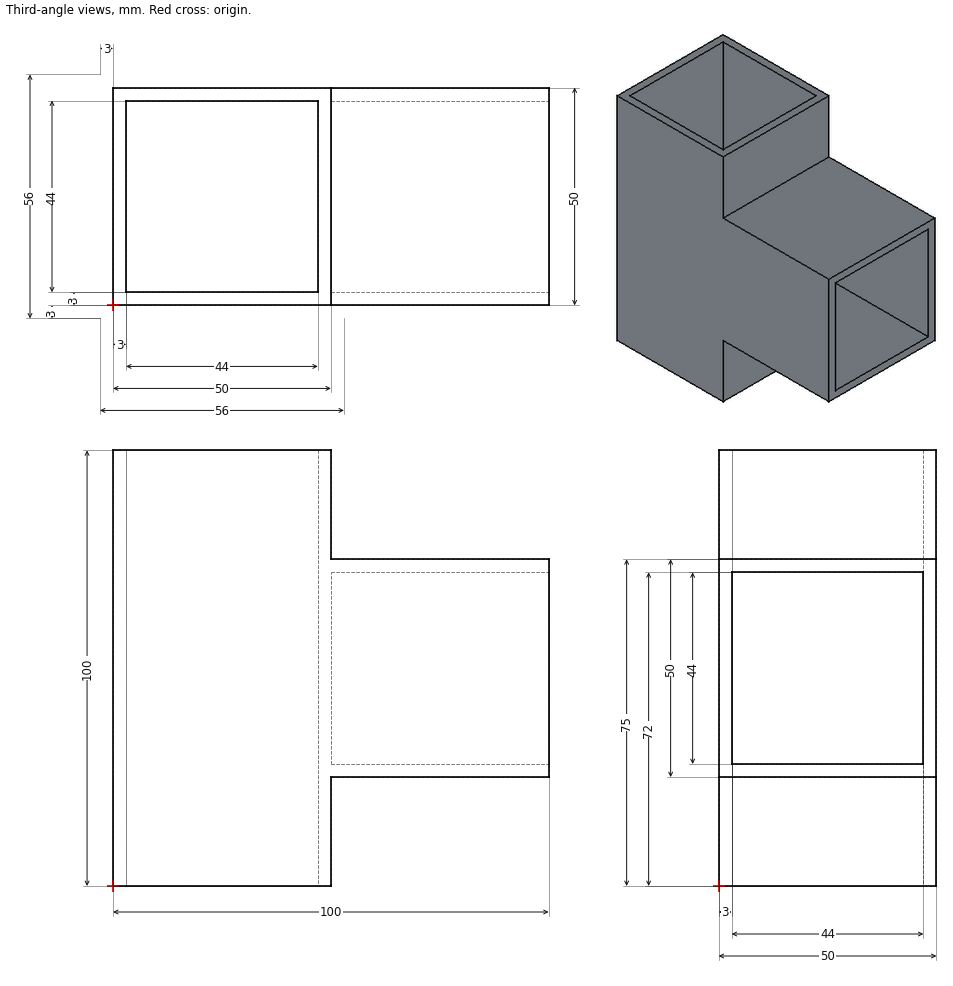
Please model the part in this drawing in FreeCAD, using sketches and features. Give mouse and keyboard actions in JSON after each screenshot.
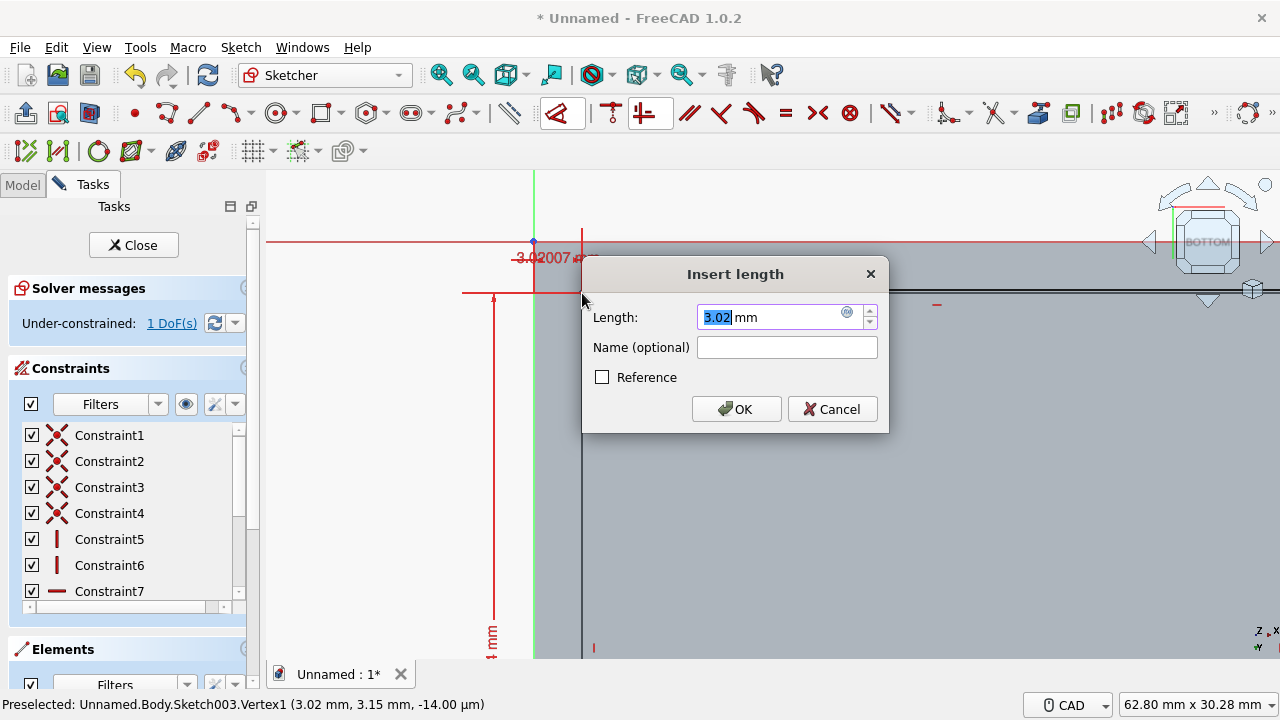
{"action": "type", "text": "3"}
{"action": "key", "text": "Return"}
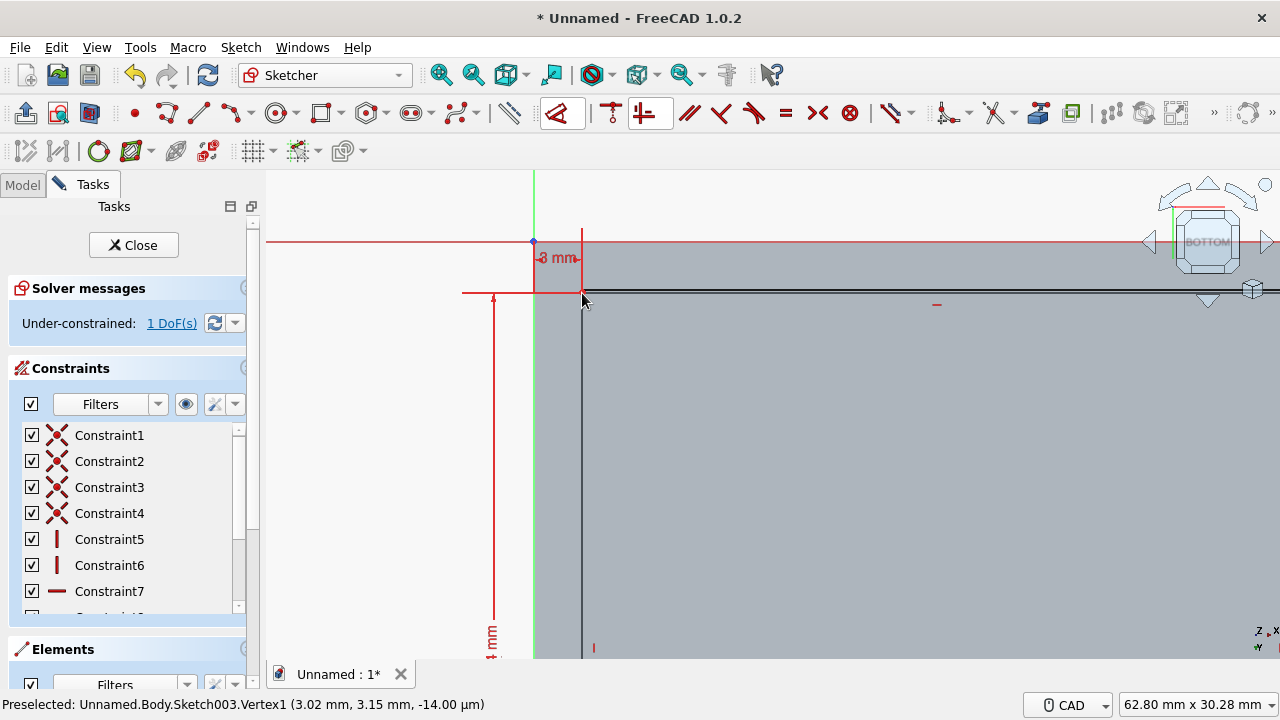
{"action": "left_click", "coordinate": [582, 293]}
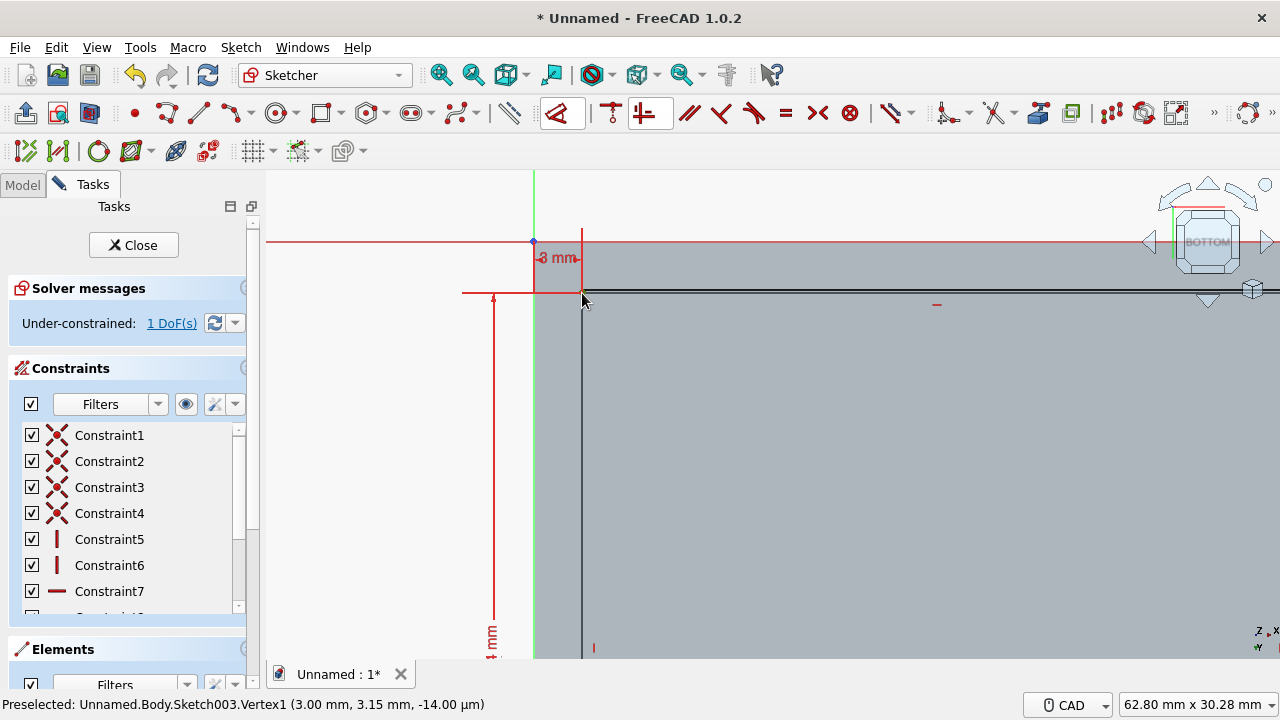
{"action": "key", "text": "i"}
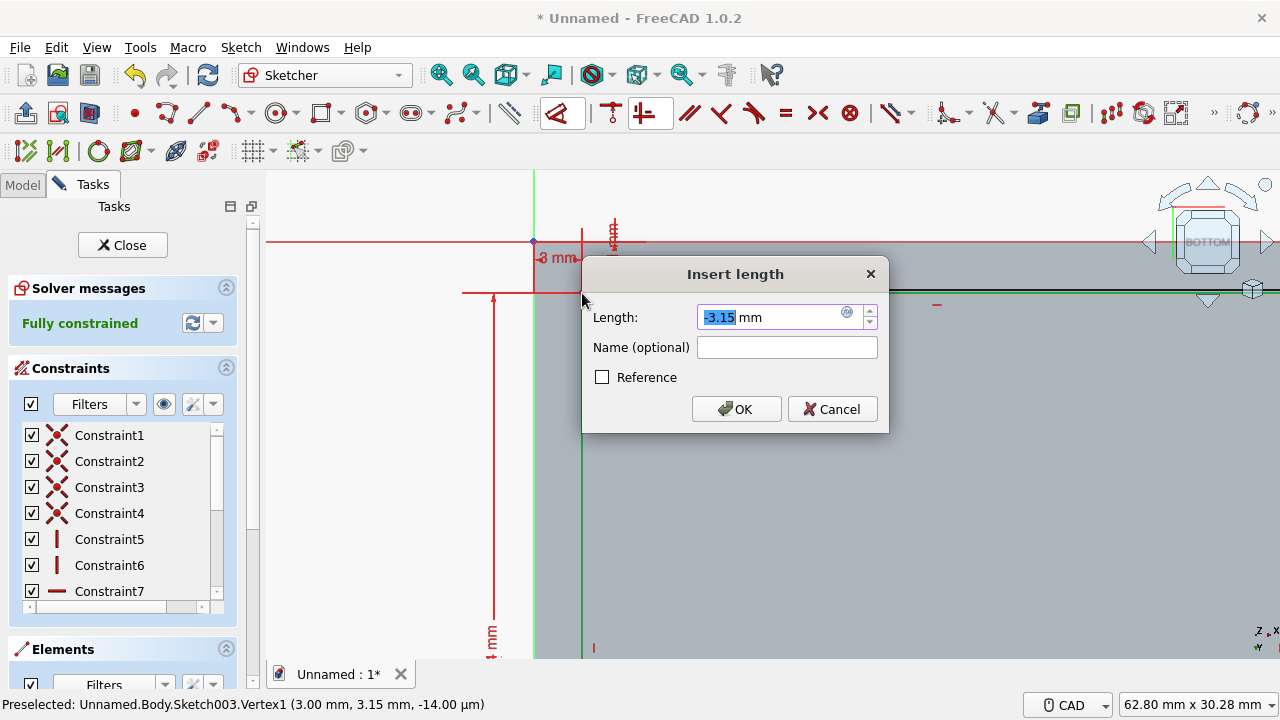
{"action": "type", "text": "-3"}
{"action": "key", "text": "Return"}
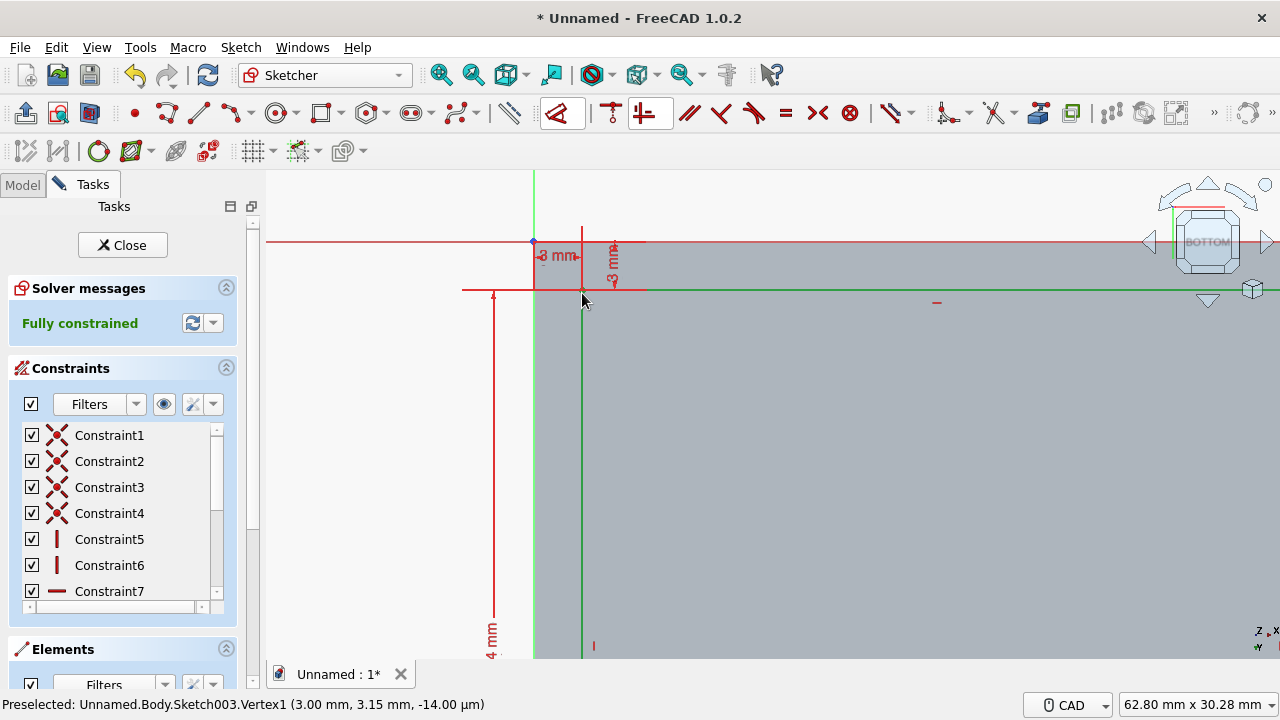
{"action": "left_click", "coordinate": [123, 245]}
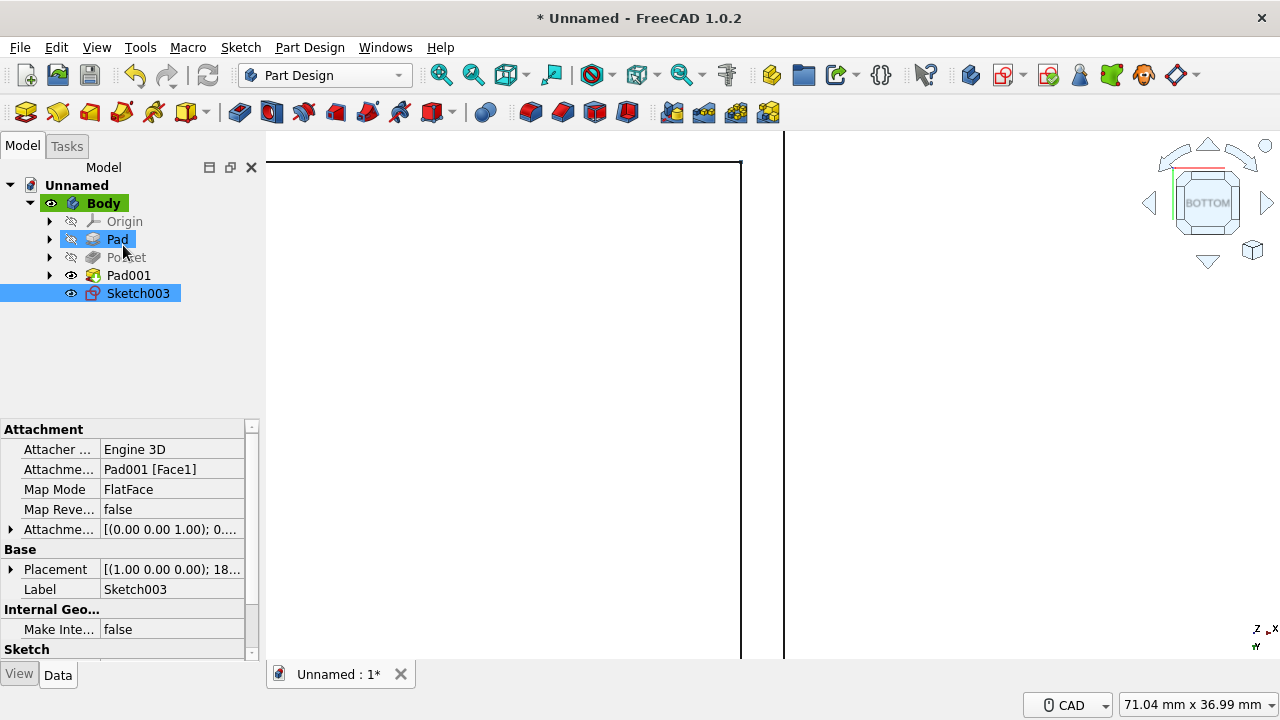
{"action": "left_click", "coordinate": [240, 112]}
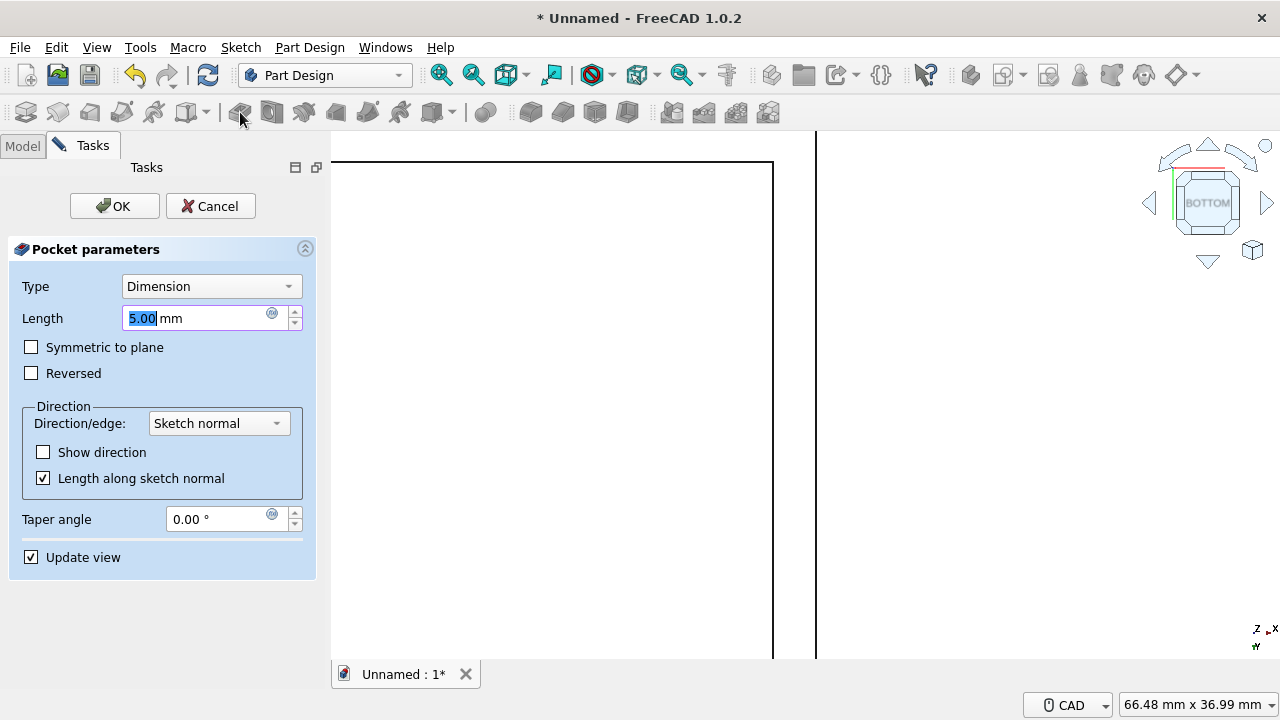
{"action": "type", "text": "100"}
{"action": "key", "text": "Tab"}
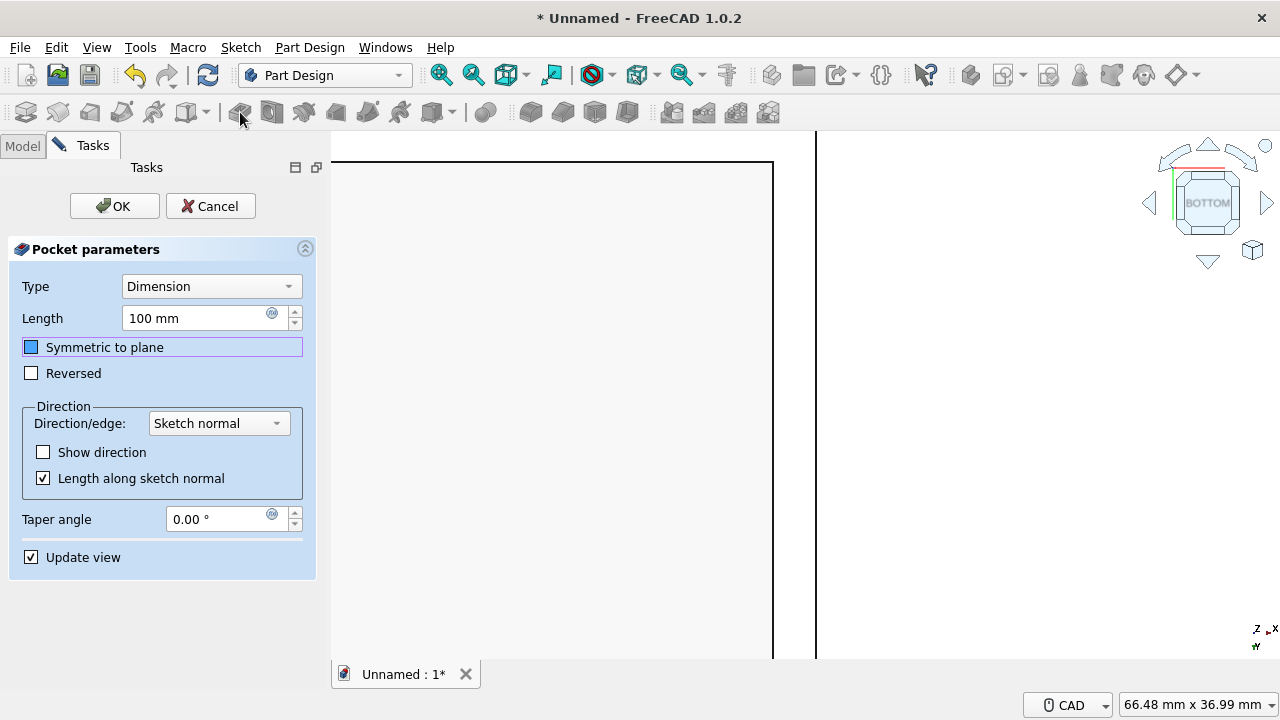
{"action": "left_click", "coordinate": [115, 206]}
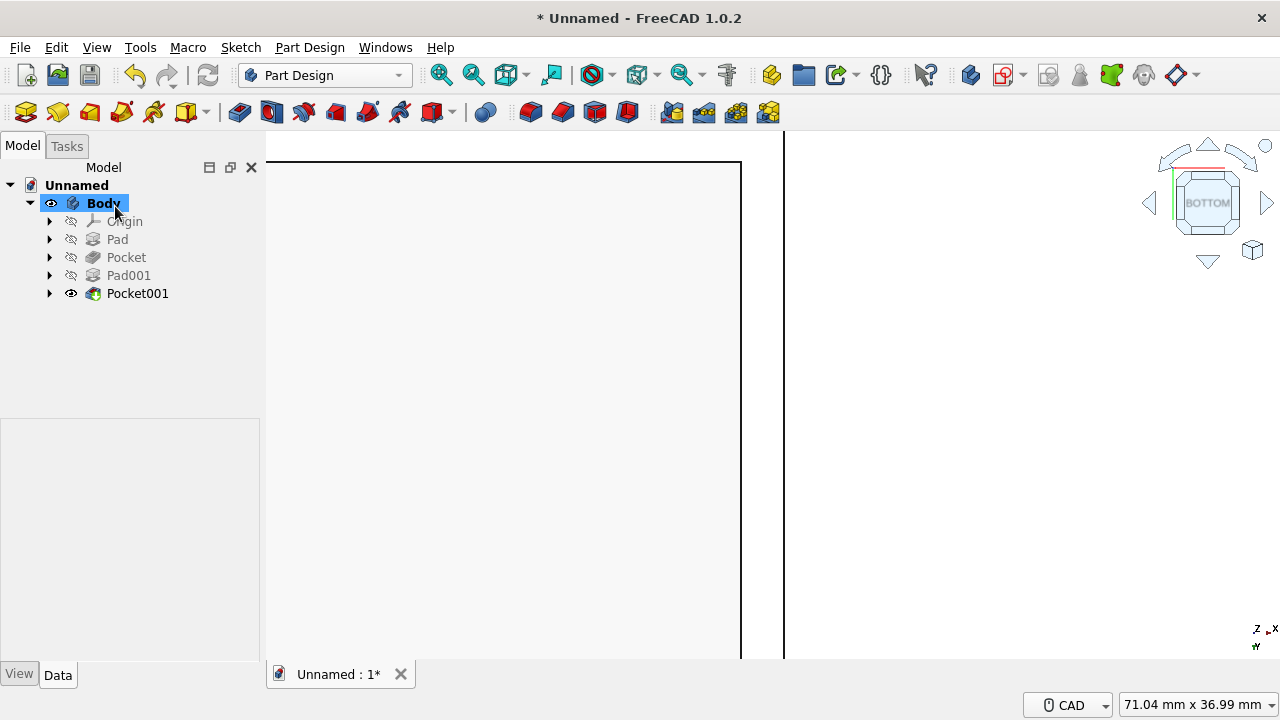
{"action": "key", "text": "0"}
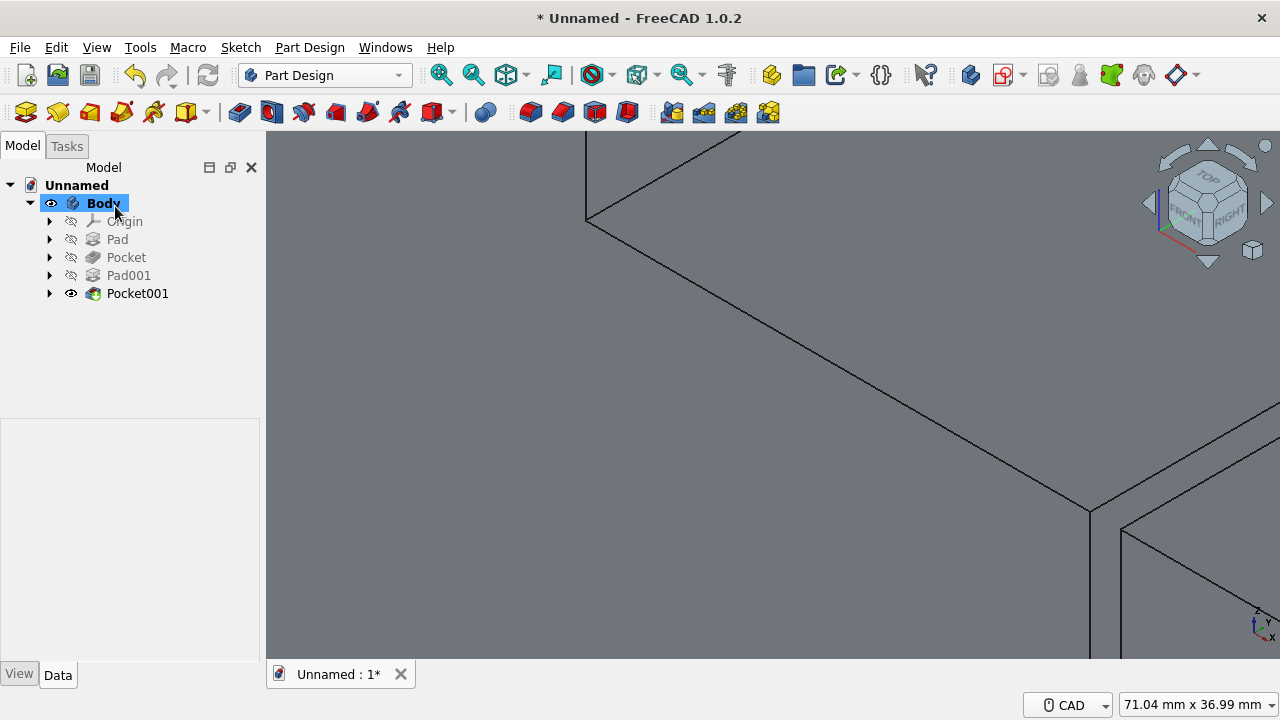
{"action": "key", "text": "v f"}